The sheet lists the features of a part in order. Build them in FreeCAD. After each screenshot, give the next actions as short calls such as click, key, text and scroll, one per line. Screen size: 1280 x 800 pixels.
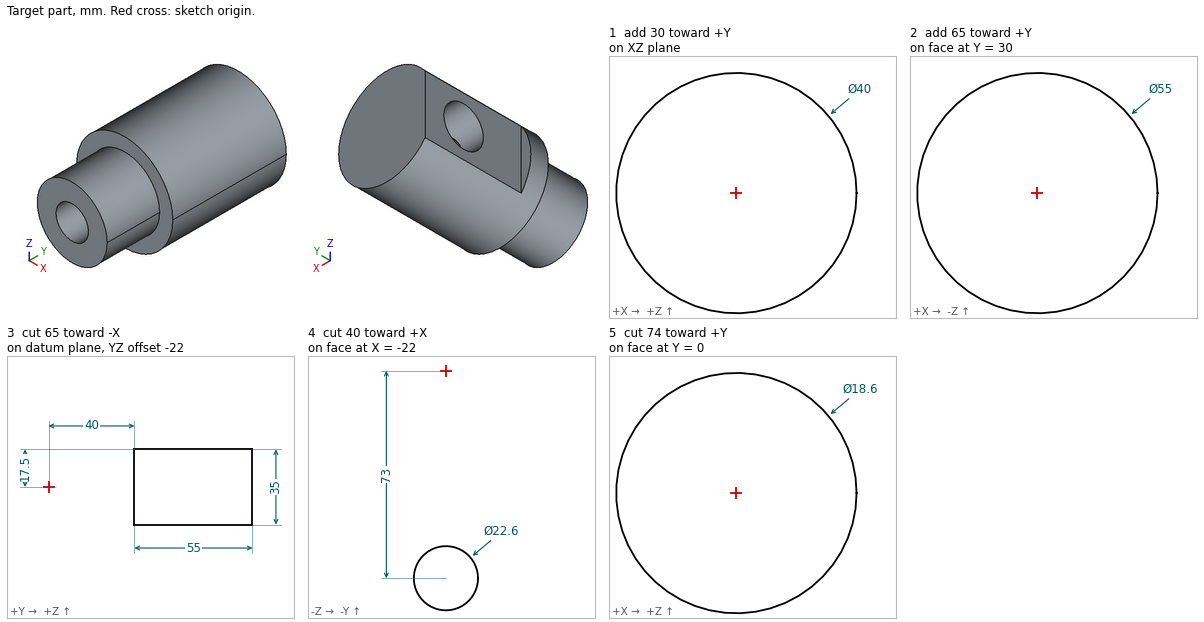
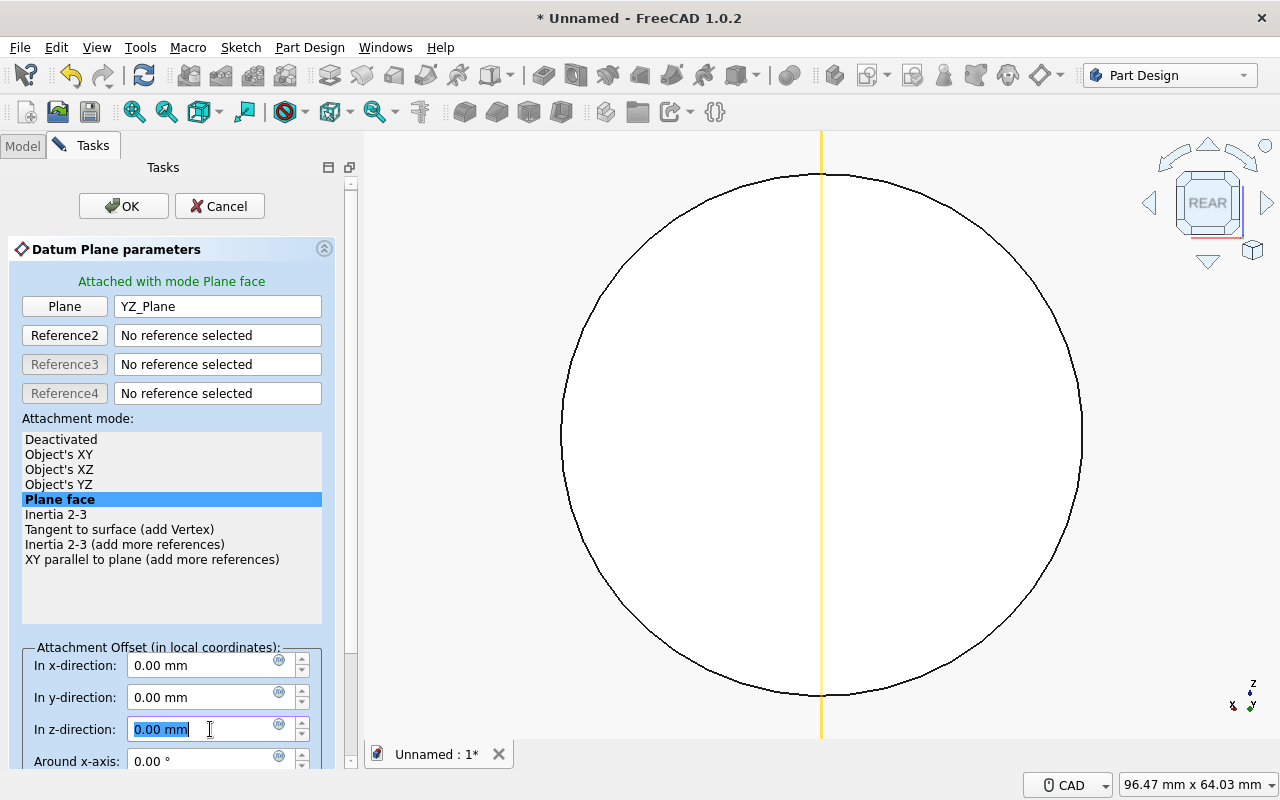
text(-22)
key(Tab)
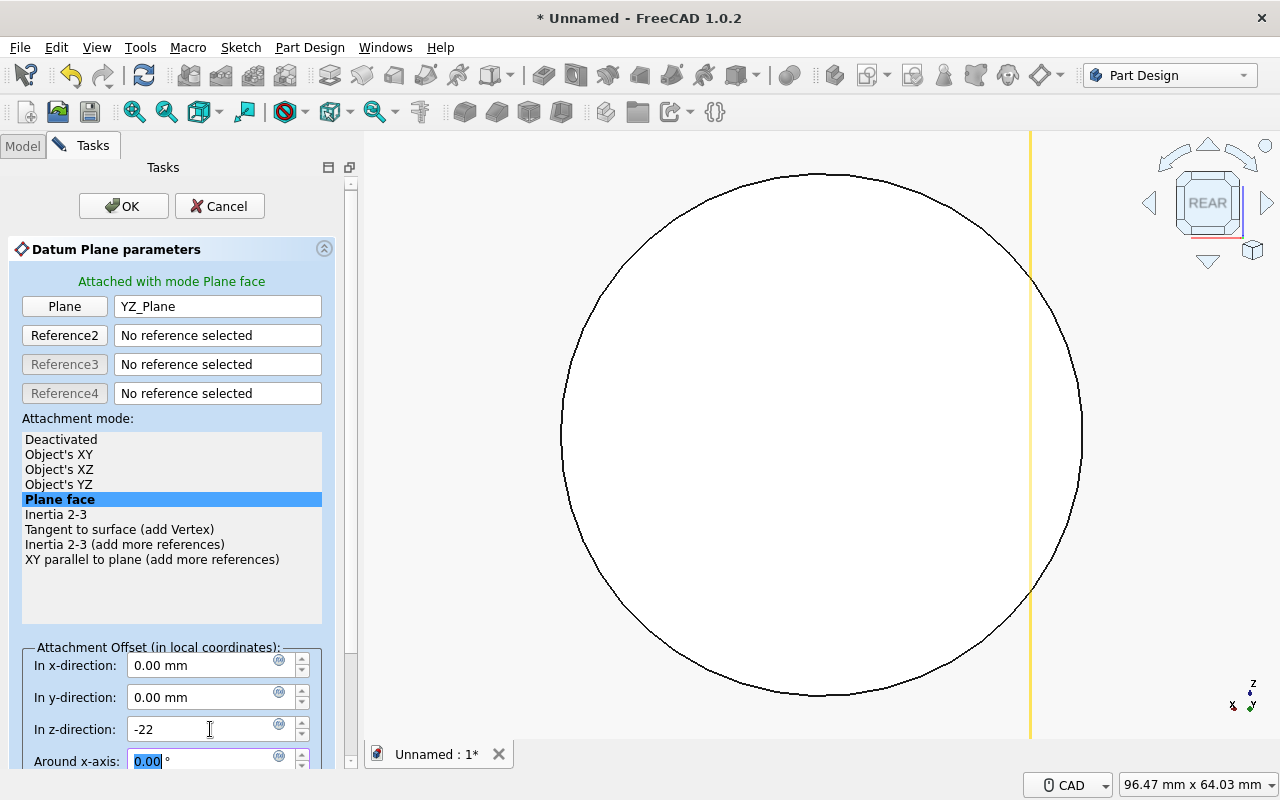
click(124, 206)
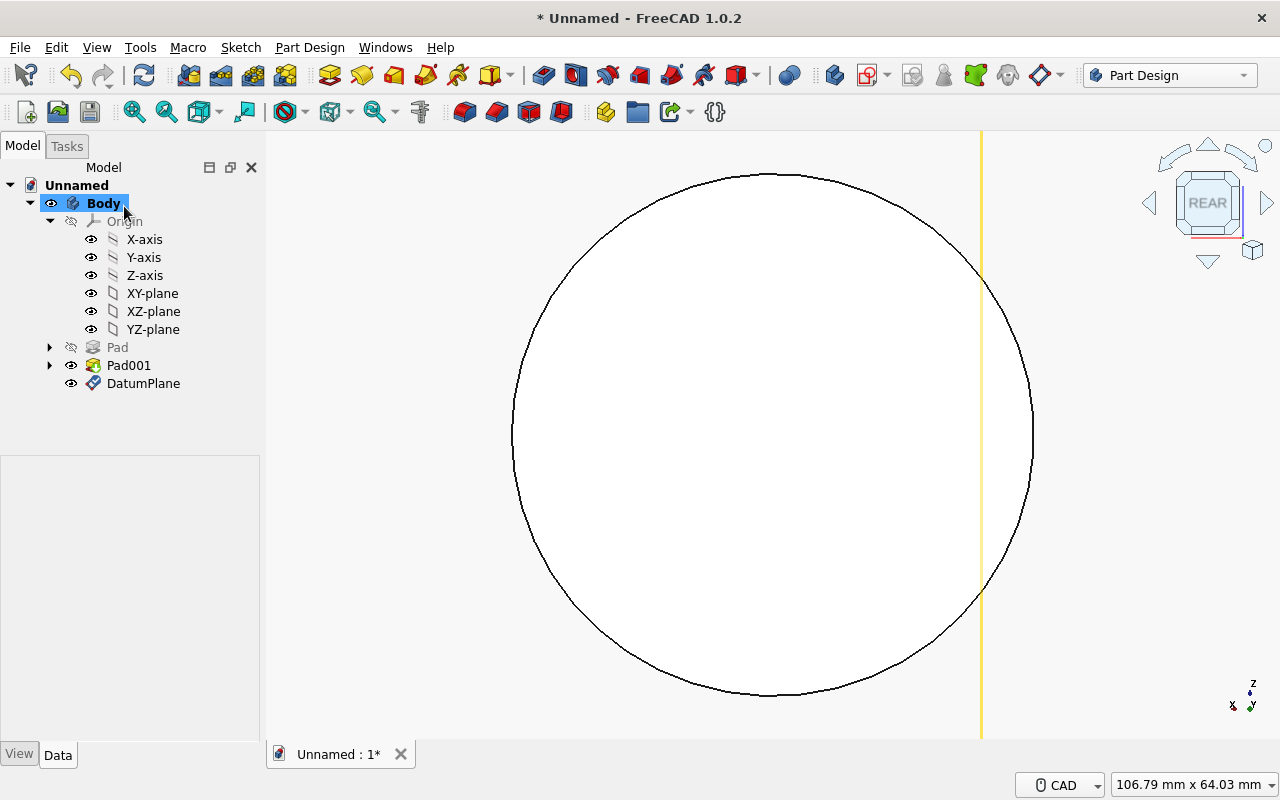
click(116, 383)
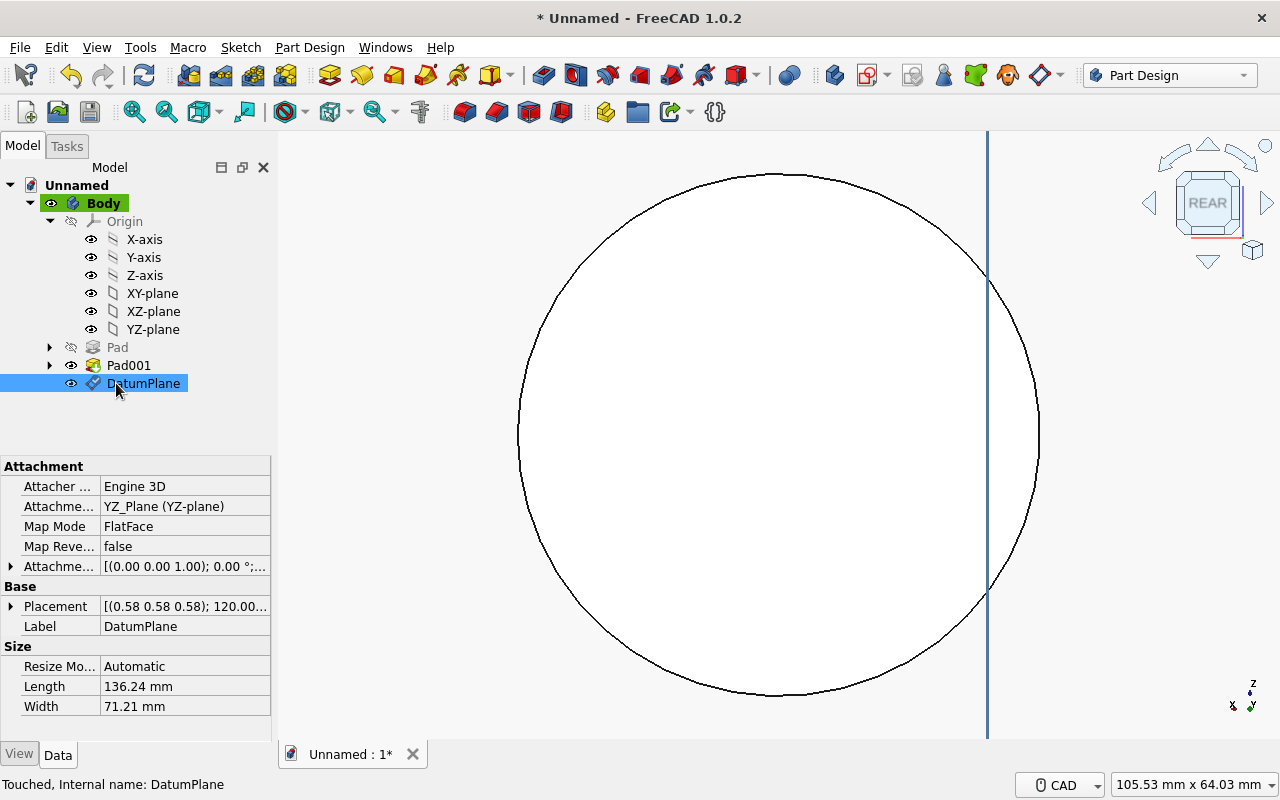
click(868, 76)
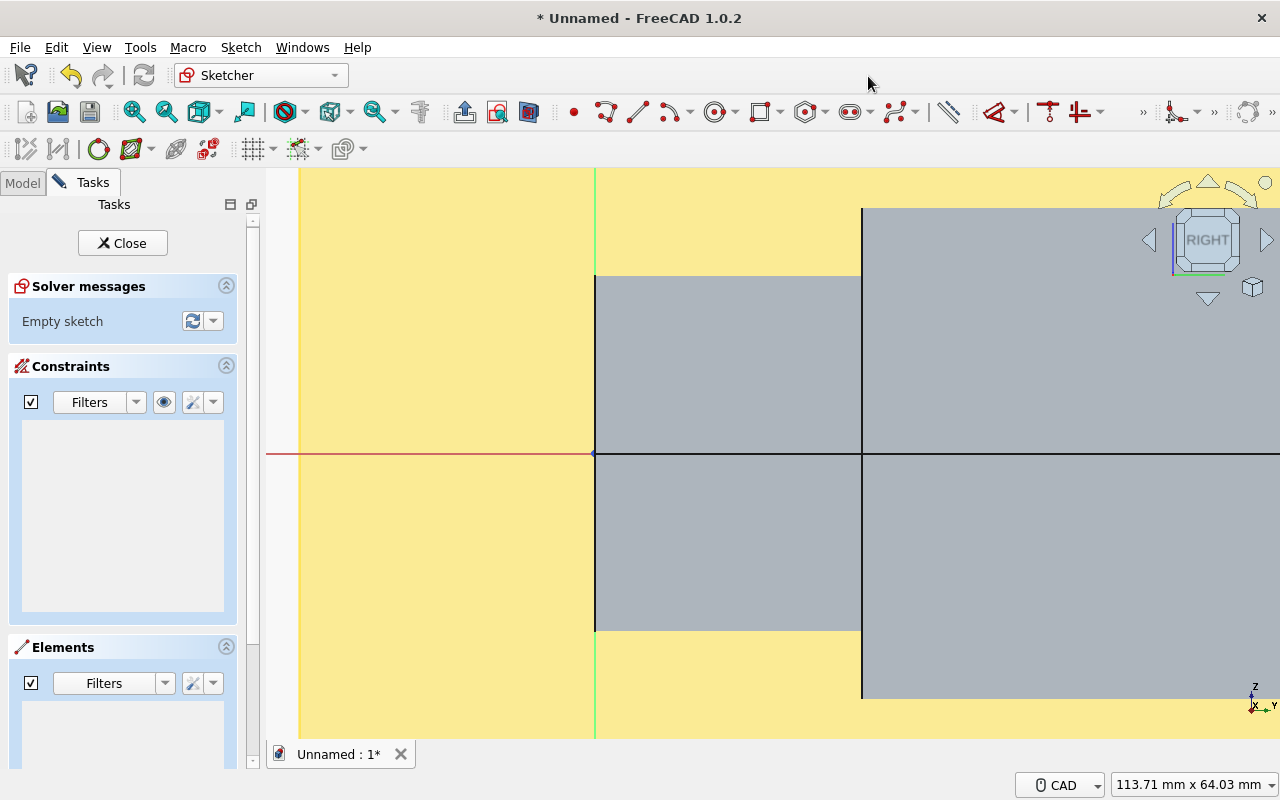
key(q)
key(s)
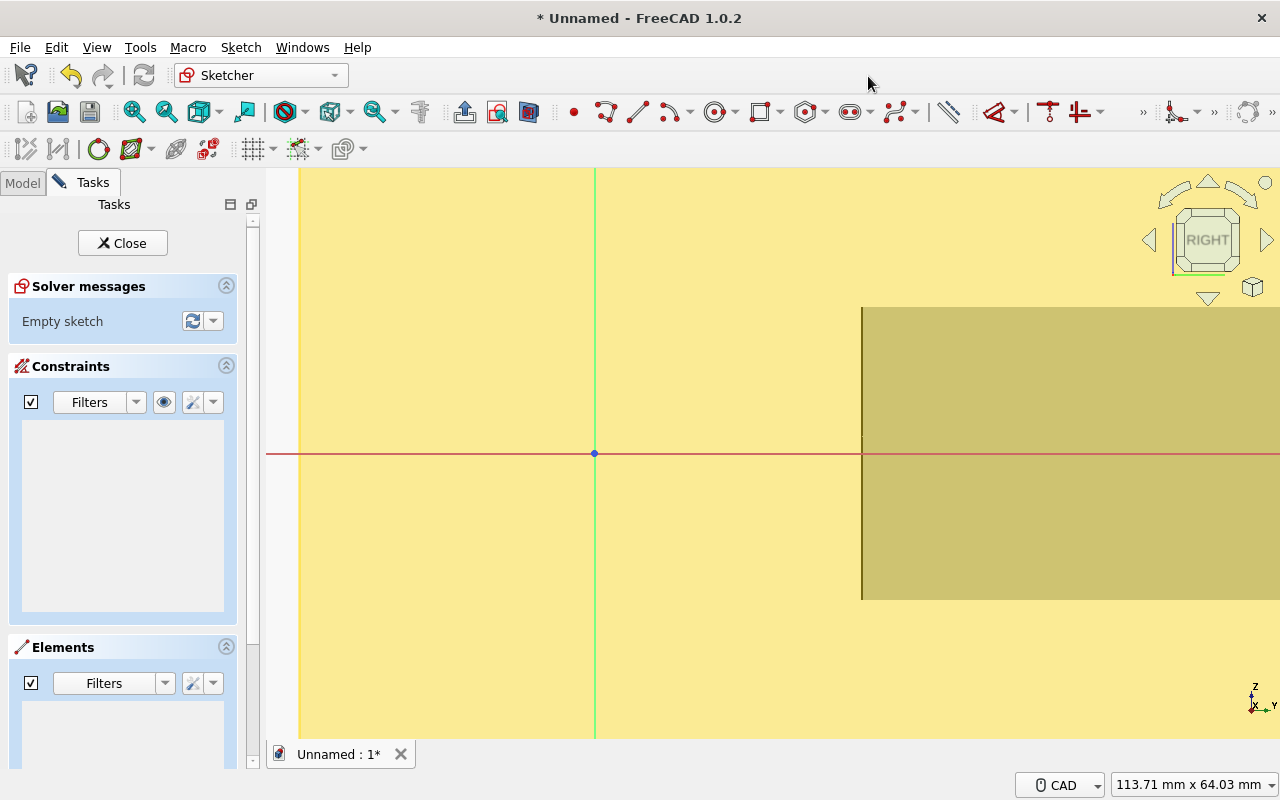
scroll(294, 453, down, 2)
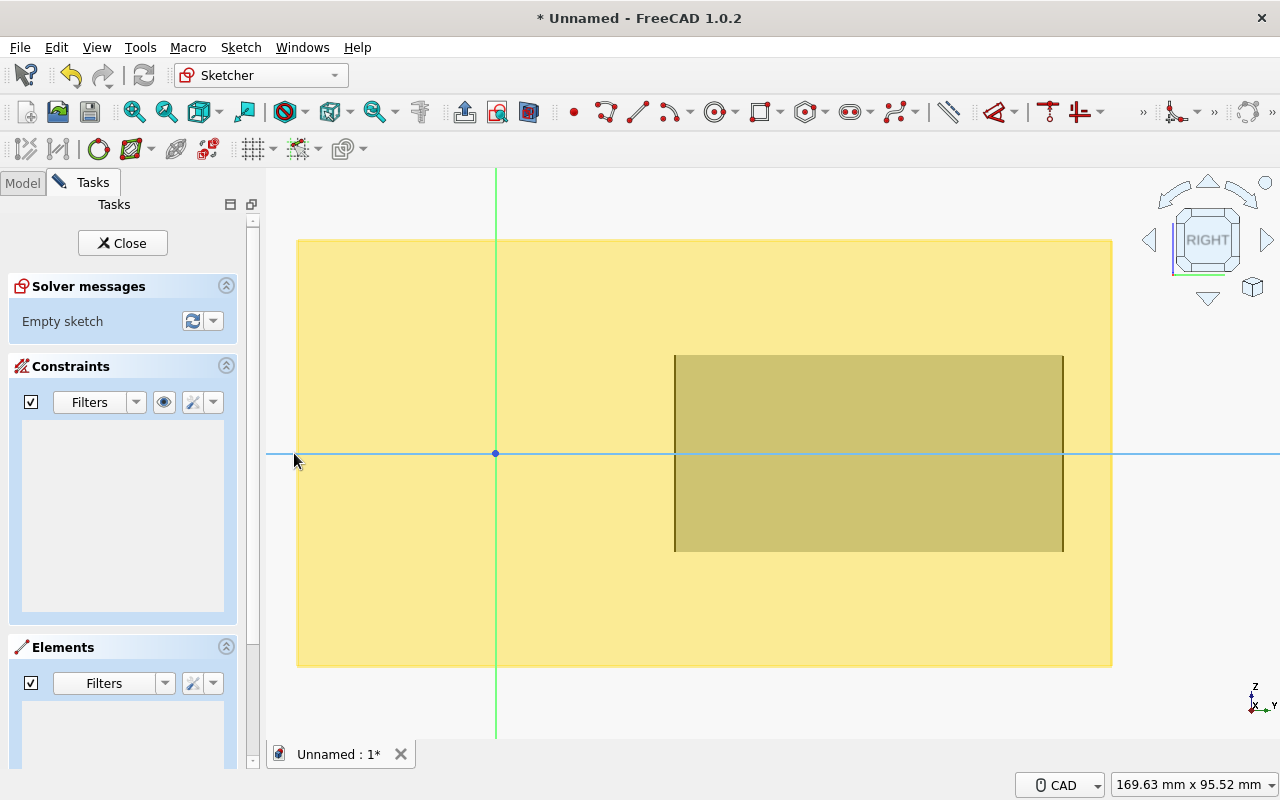
click(760, 112)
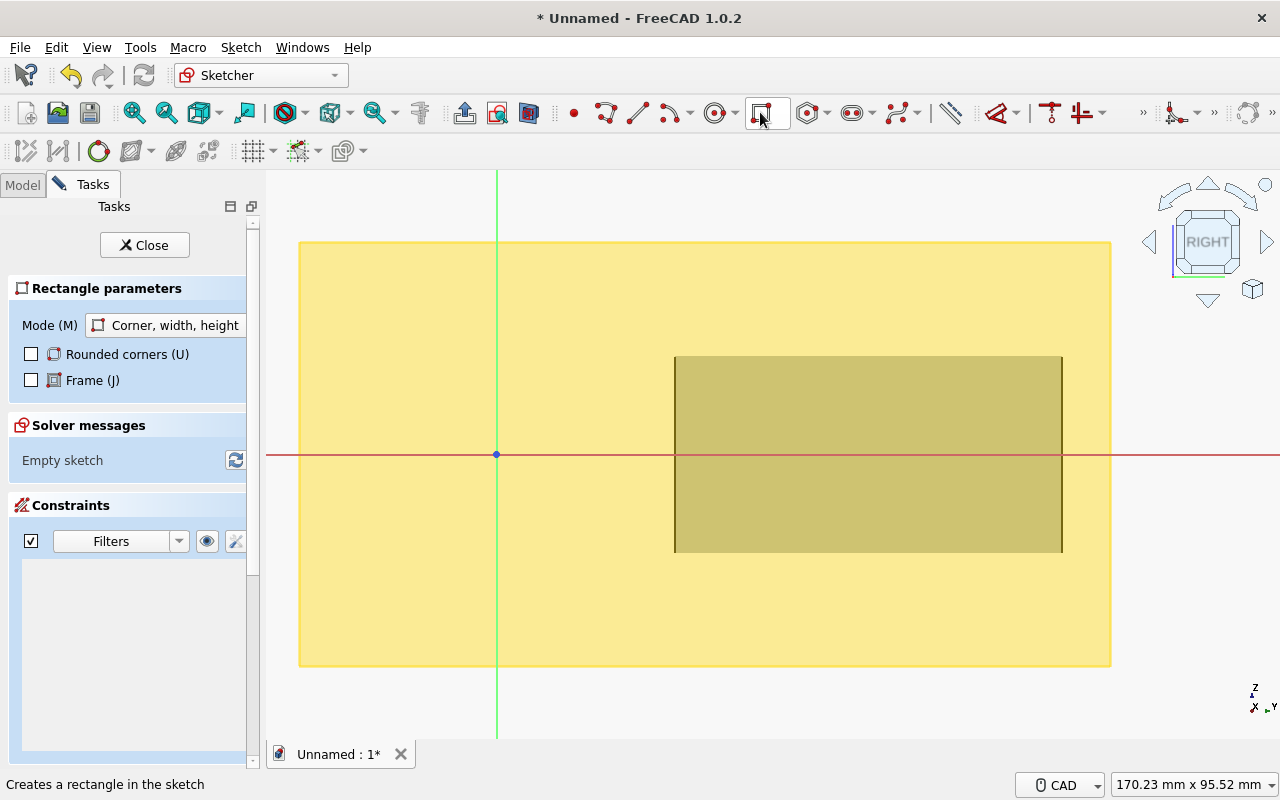
click(735, 350)
move(1062, 559)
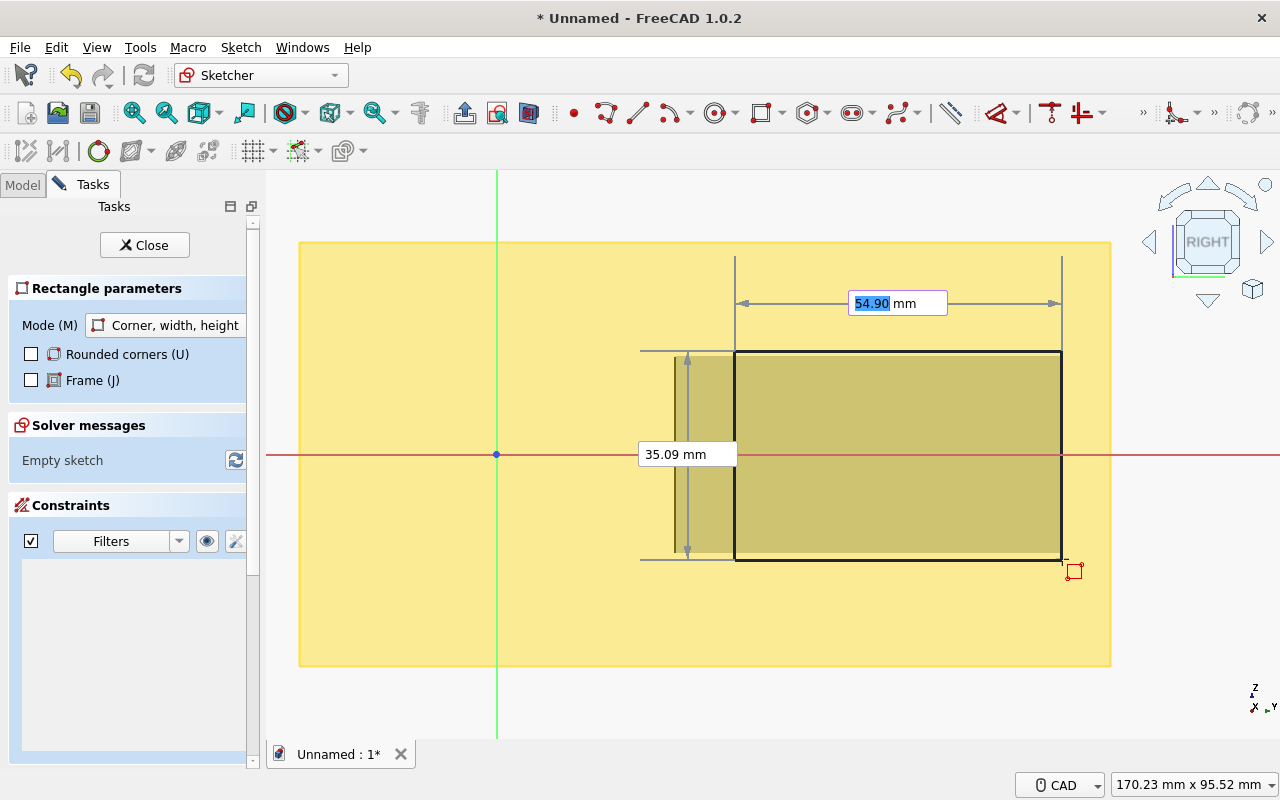
text(55)
key(Tab)
text(35)
key(Return)
key(Escape)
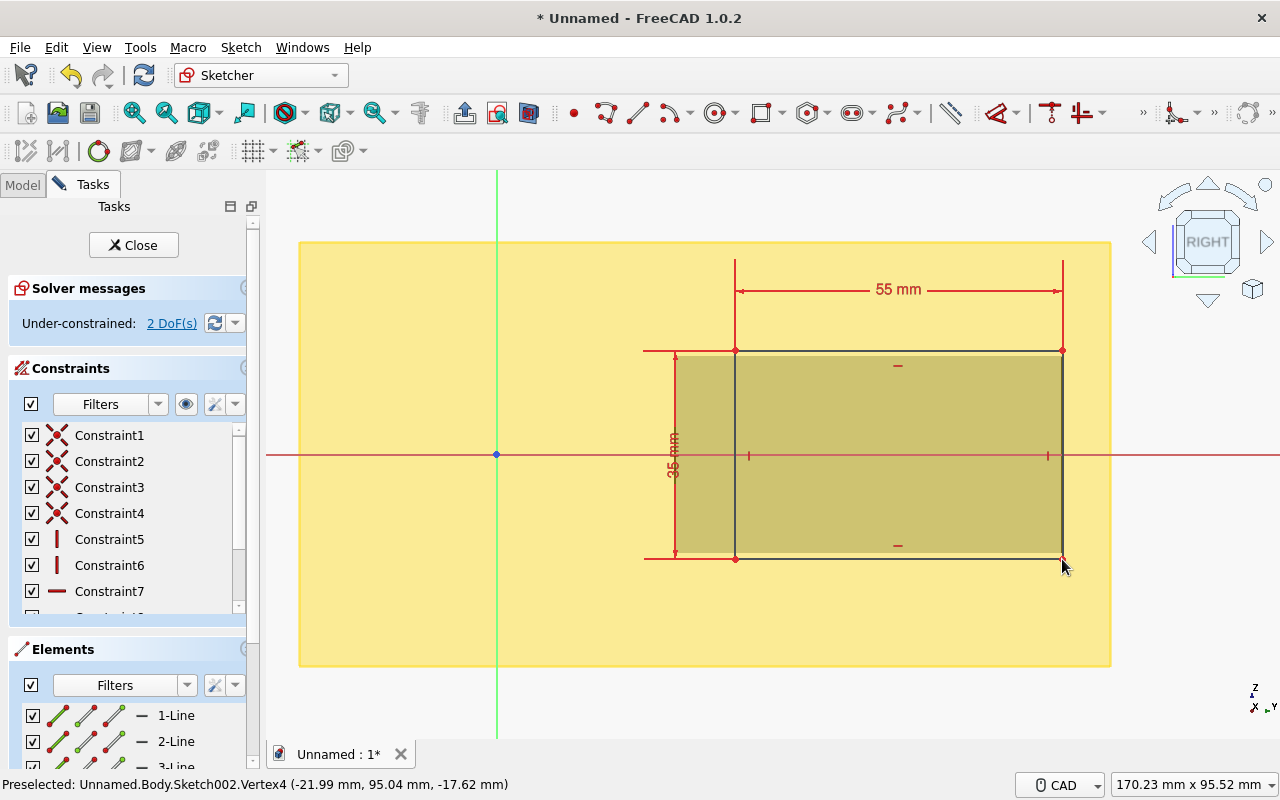
click(996, 114)